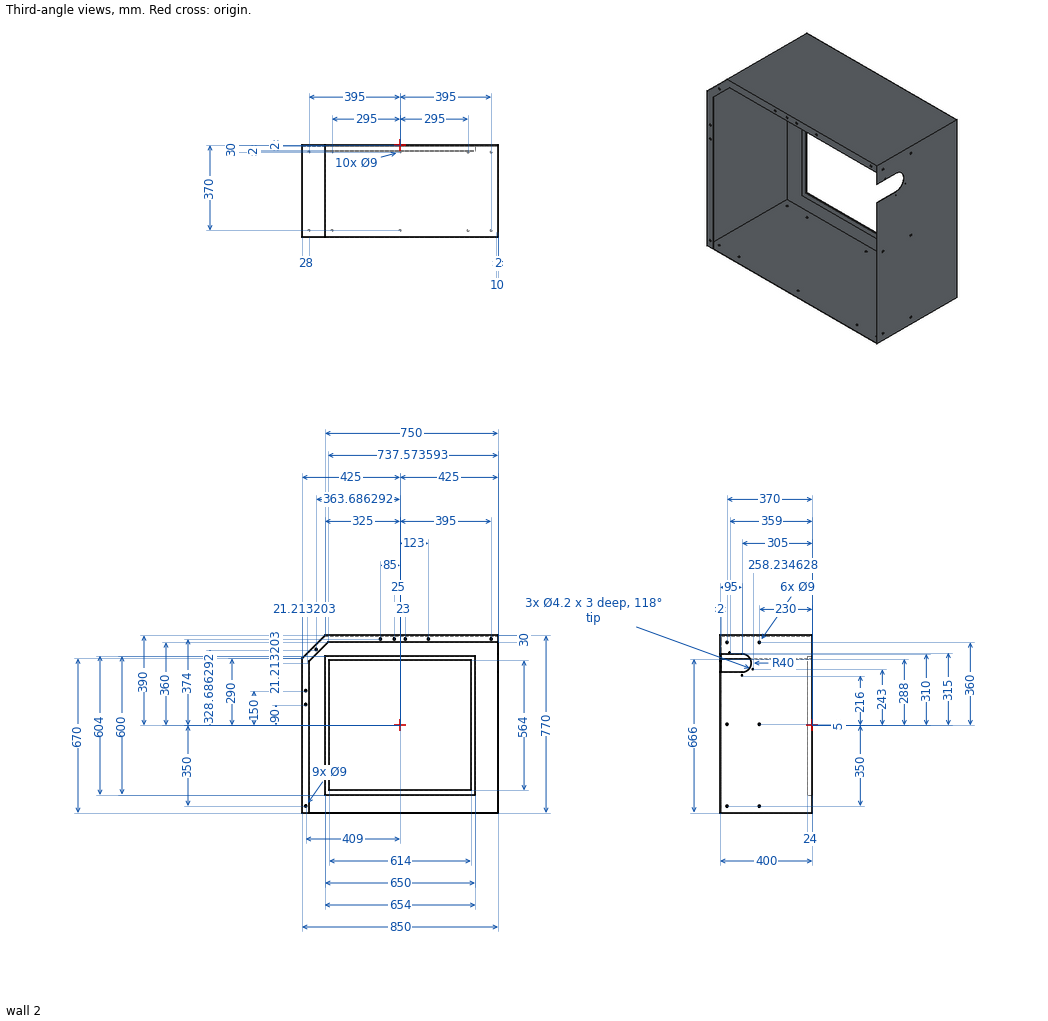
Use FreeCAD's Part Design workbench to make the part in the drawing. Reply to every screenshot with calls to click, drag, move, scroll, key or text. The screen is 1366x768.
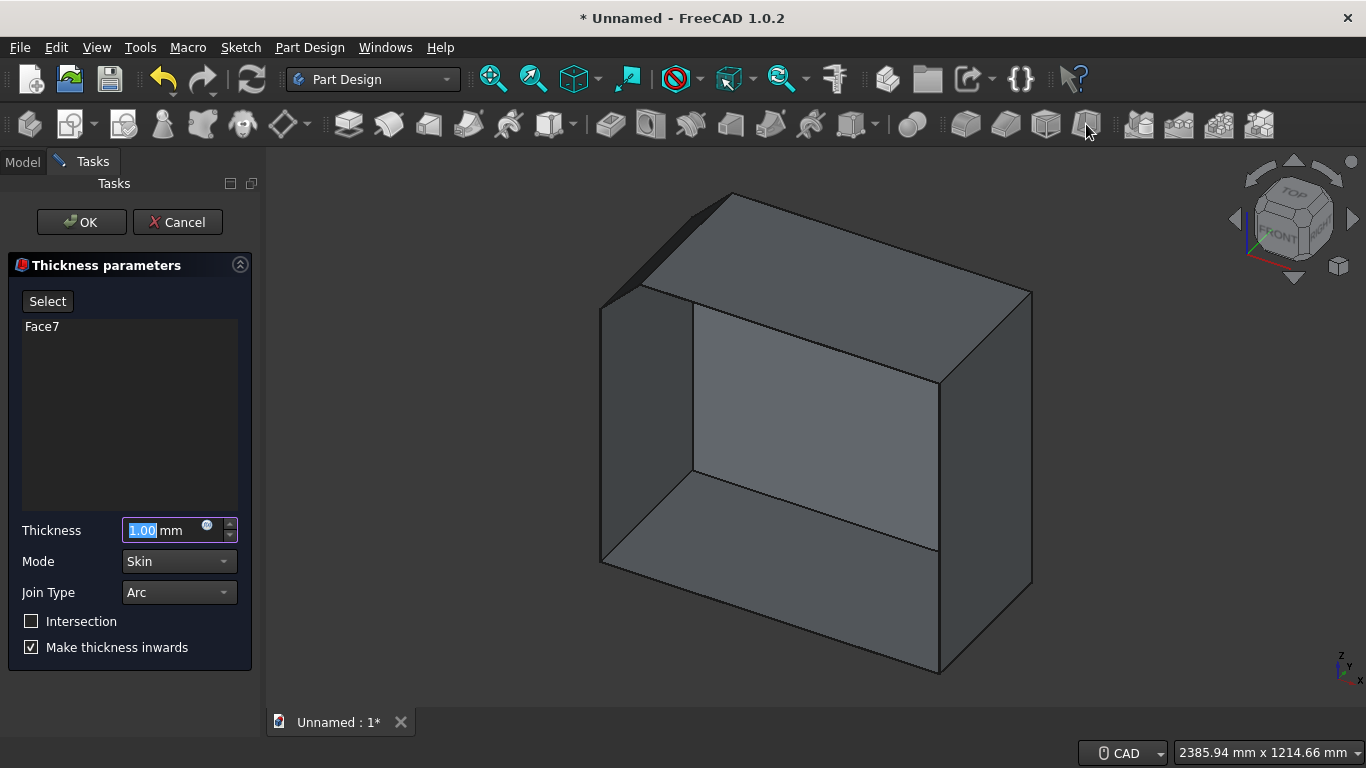
text(2)
key(Tab)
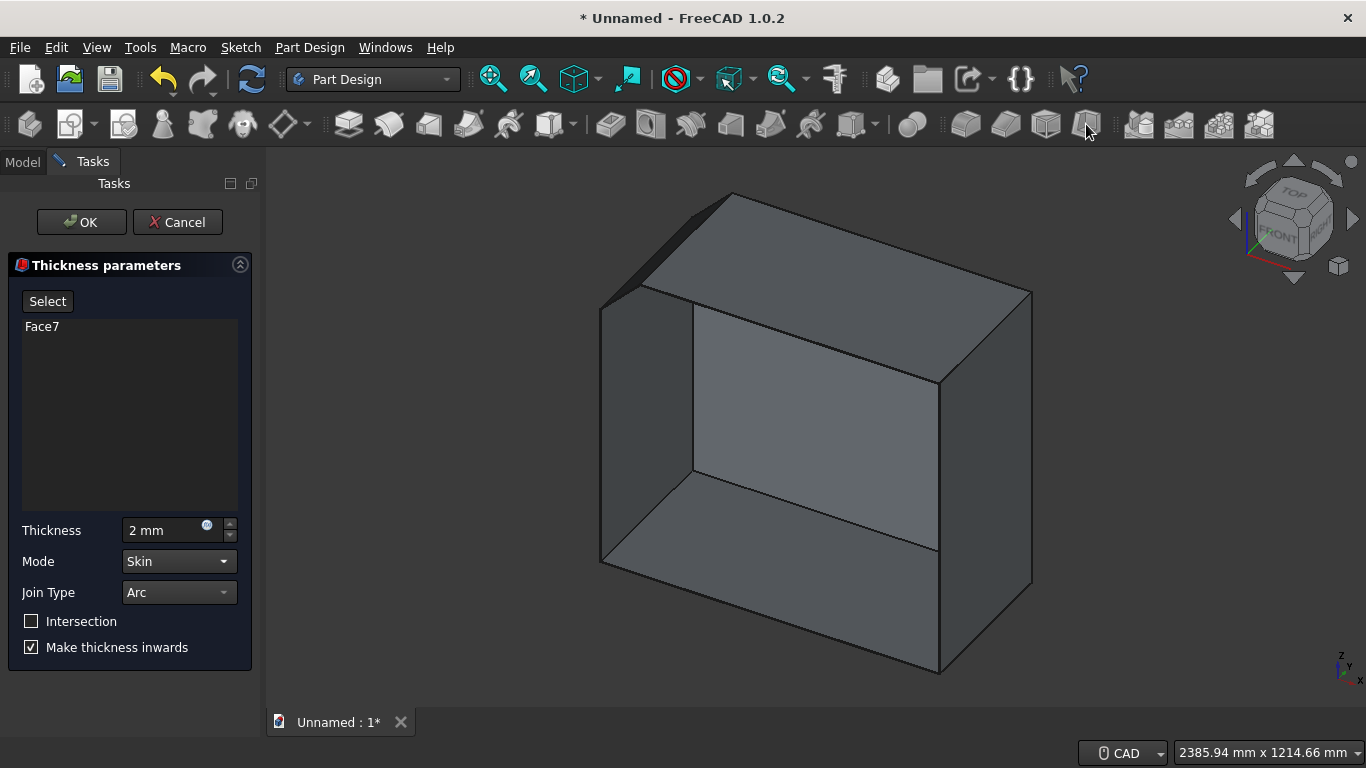
click(180, 592)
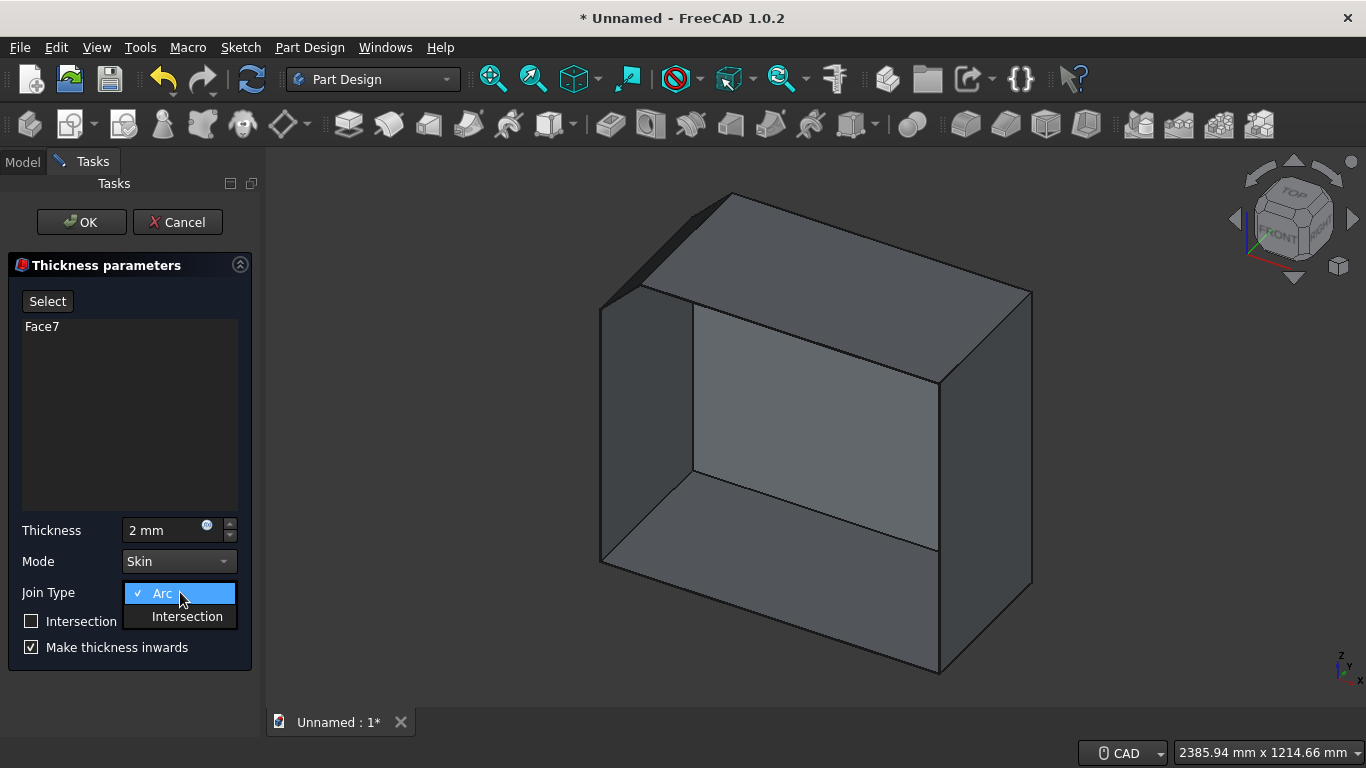
click(179, 616)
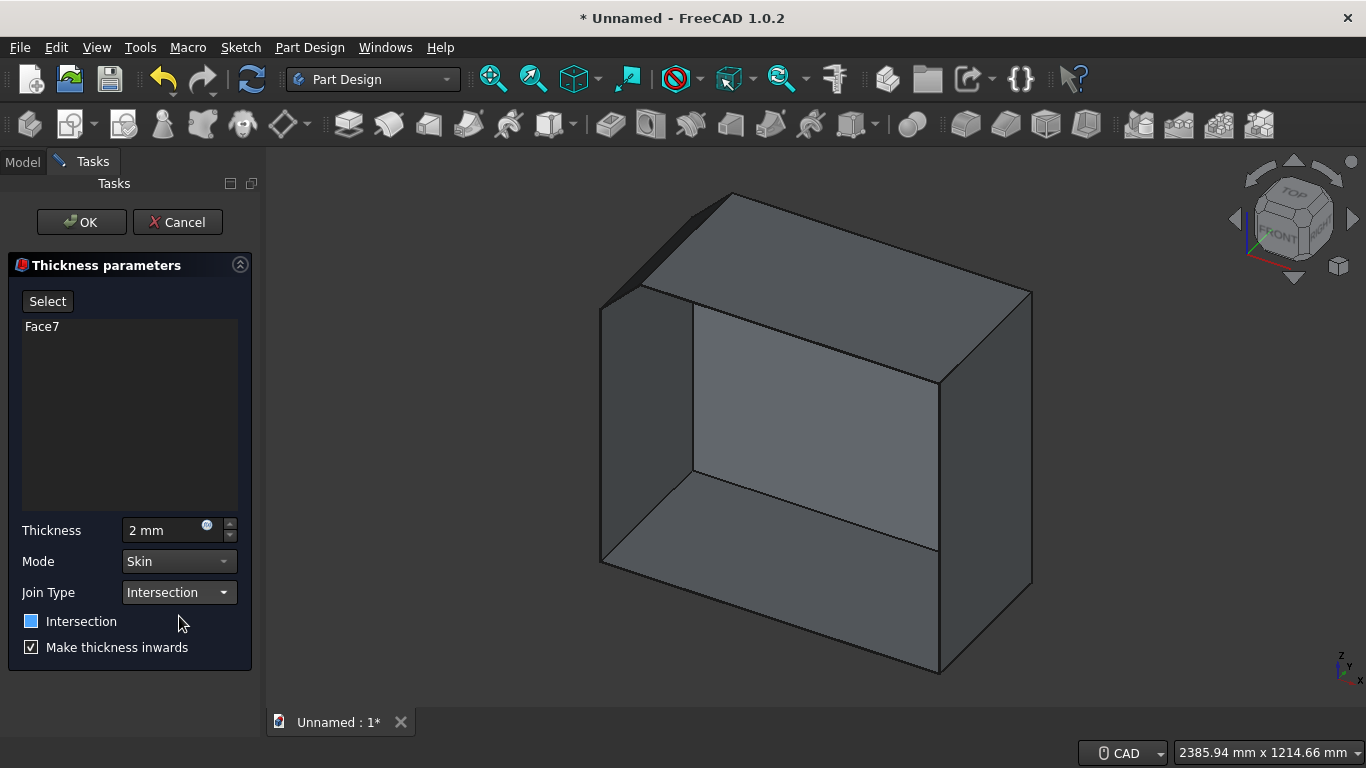
click(82, 222)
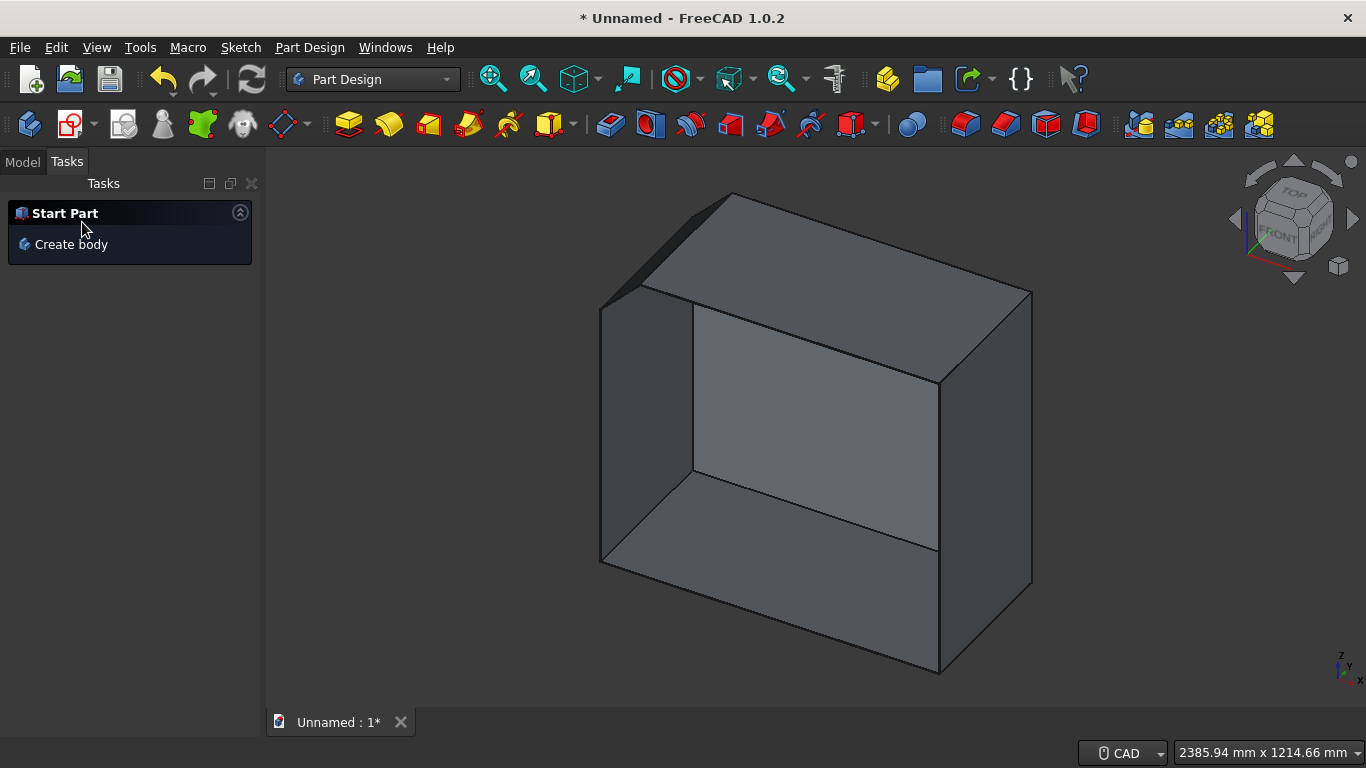
key(4)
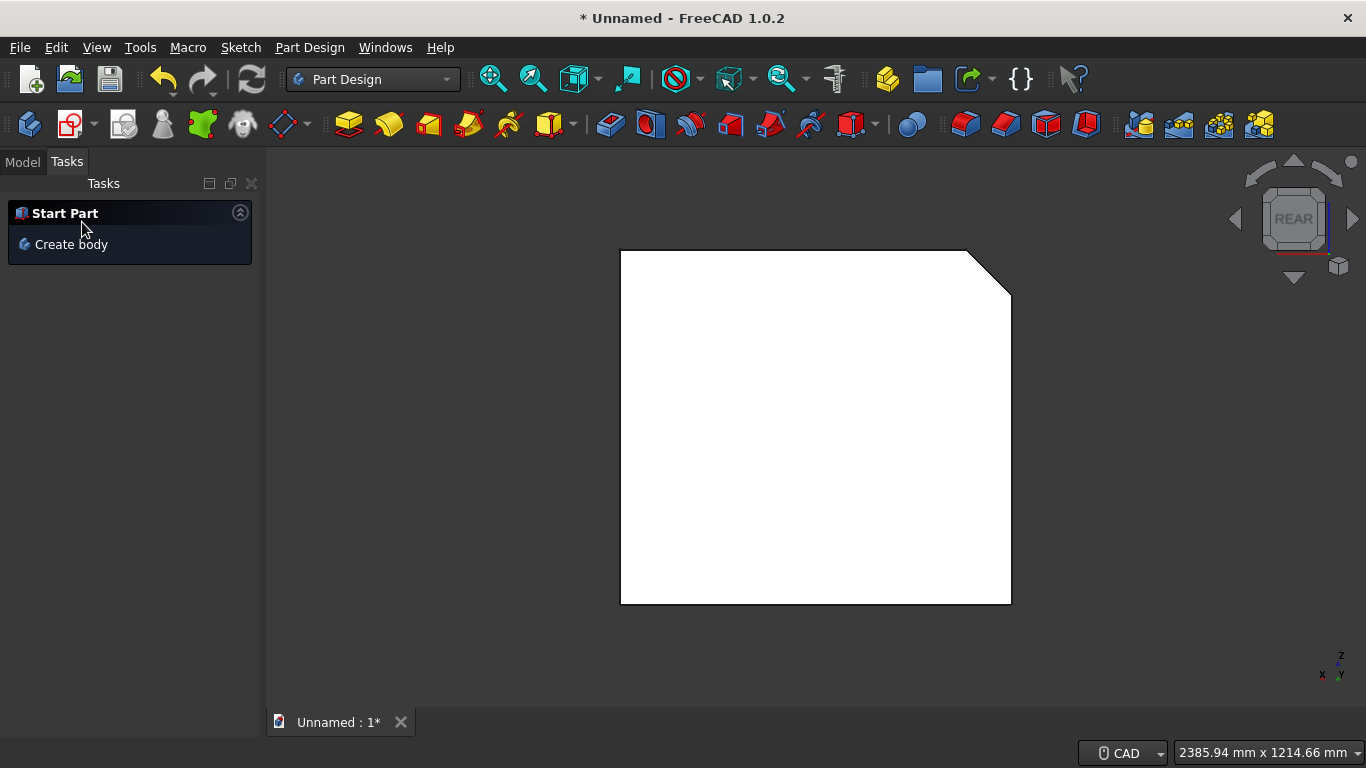
click(816, 426)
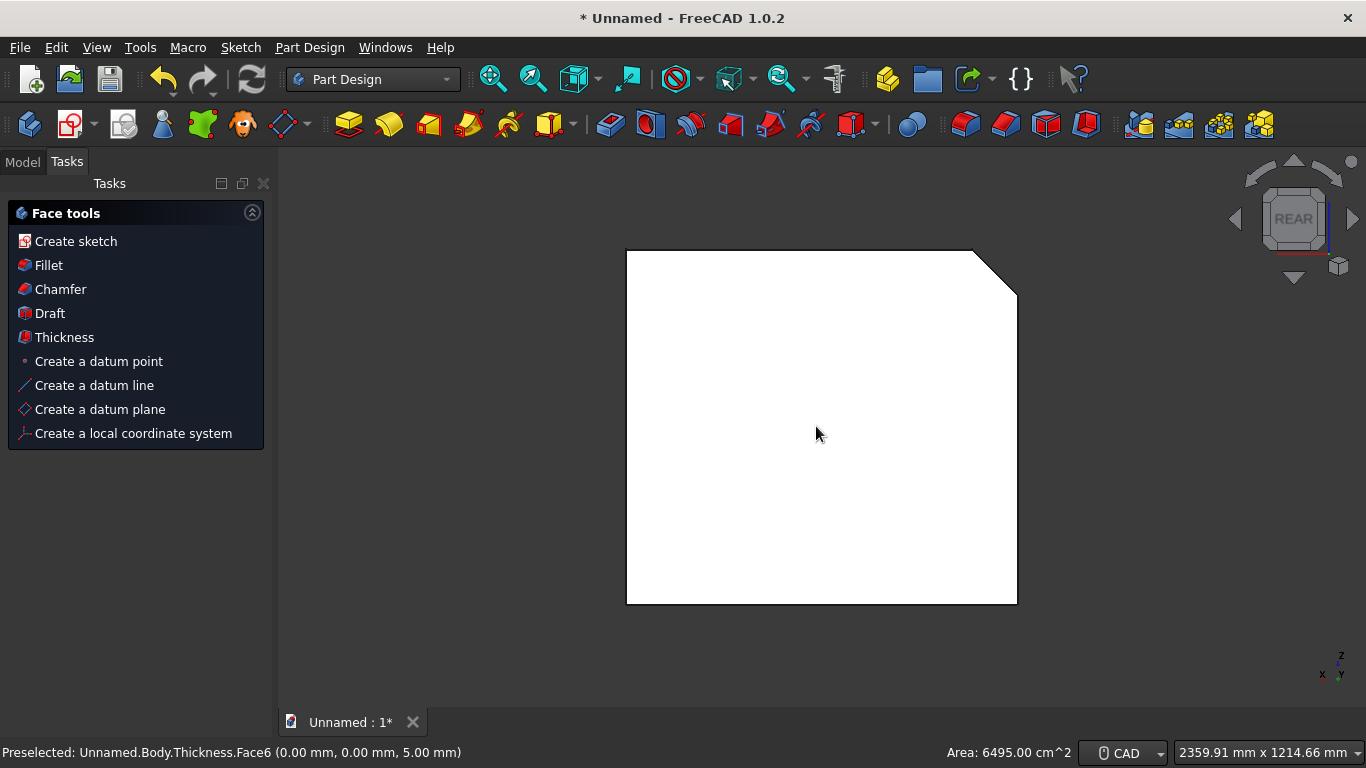
click(70, 124)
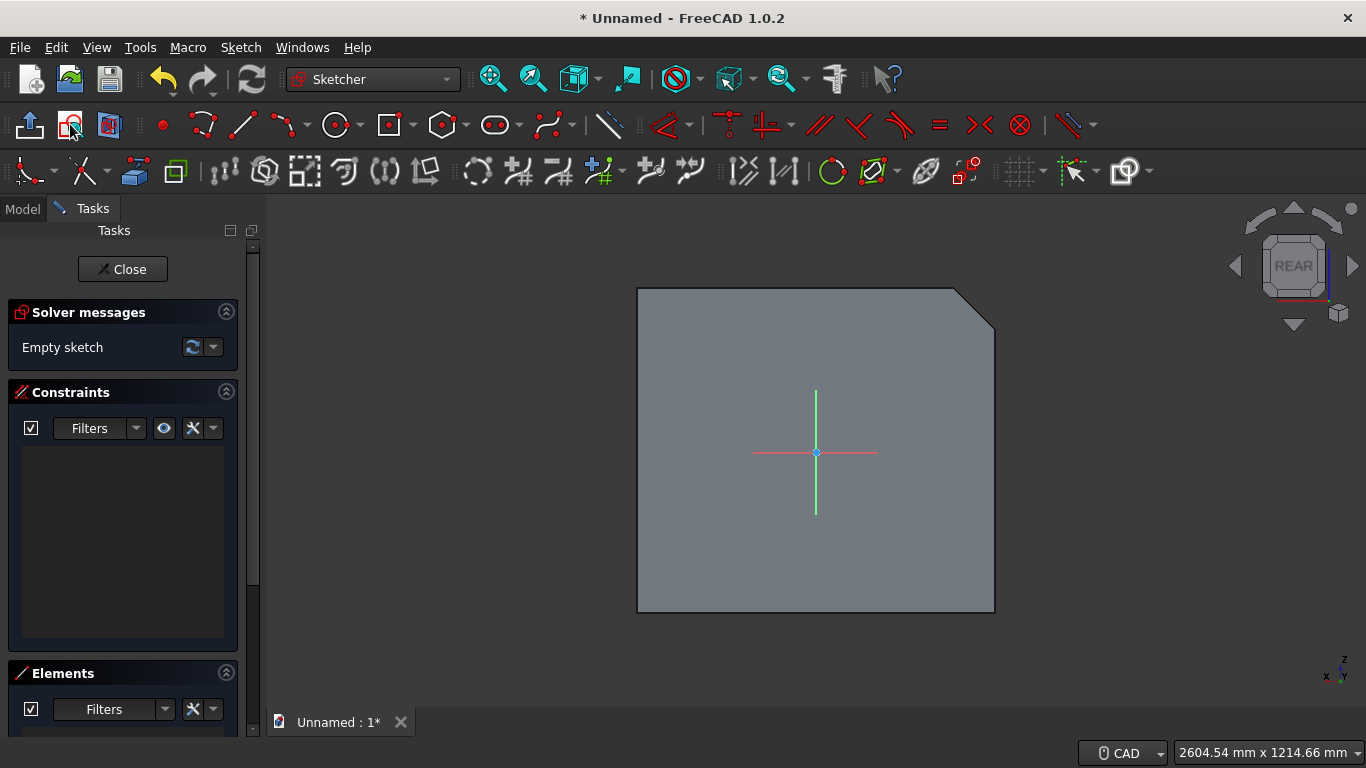
click(390, 126)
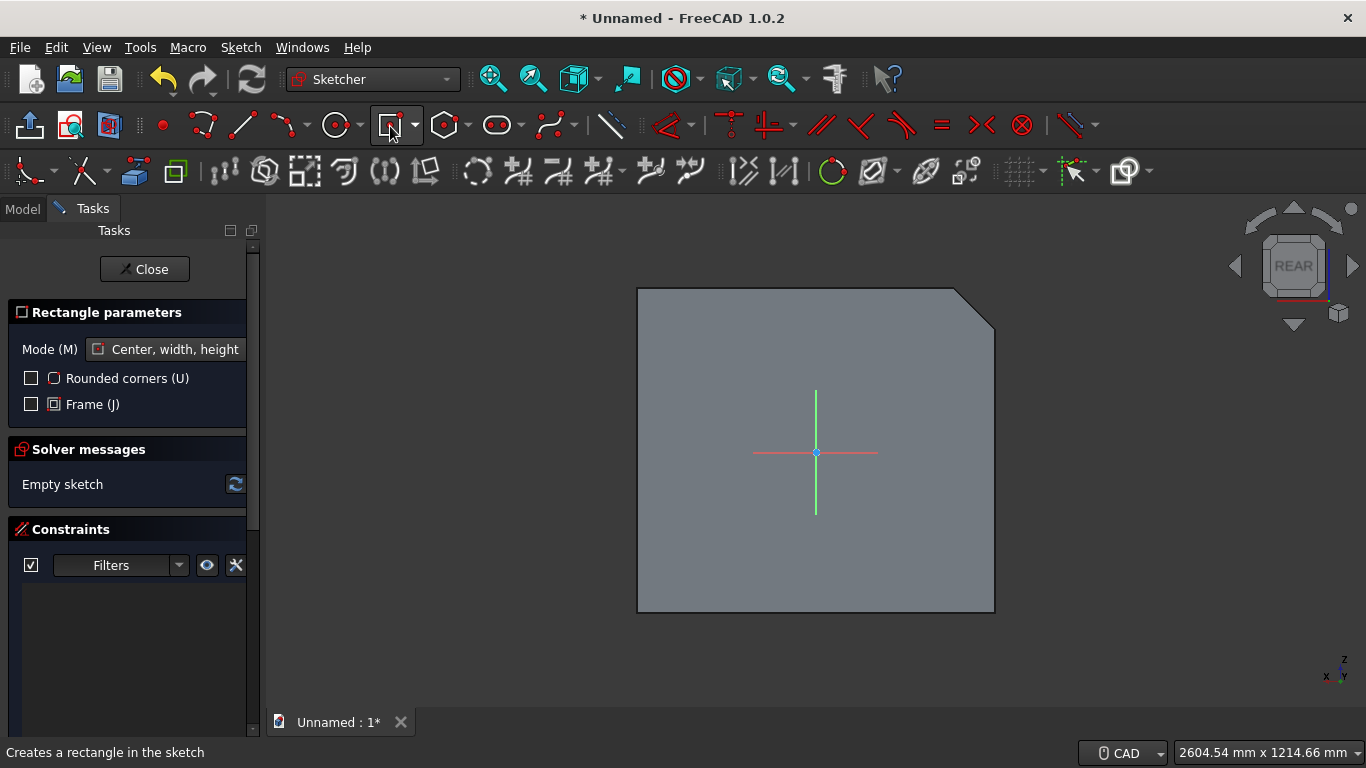
click(816, 453)
move(953, 326)